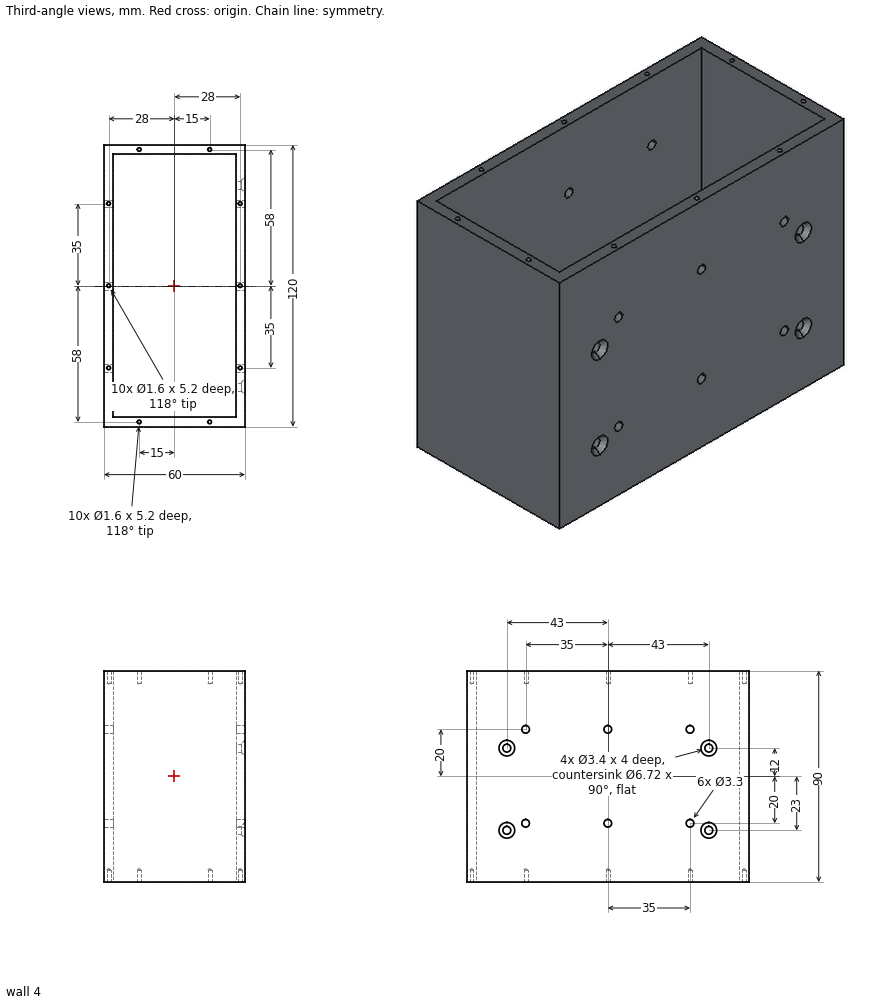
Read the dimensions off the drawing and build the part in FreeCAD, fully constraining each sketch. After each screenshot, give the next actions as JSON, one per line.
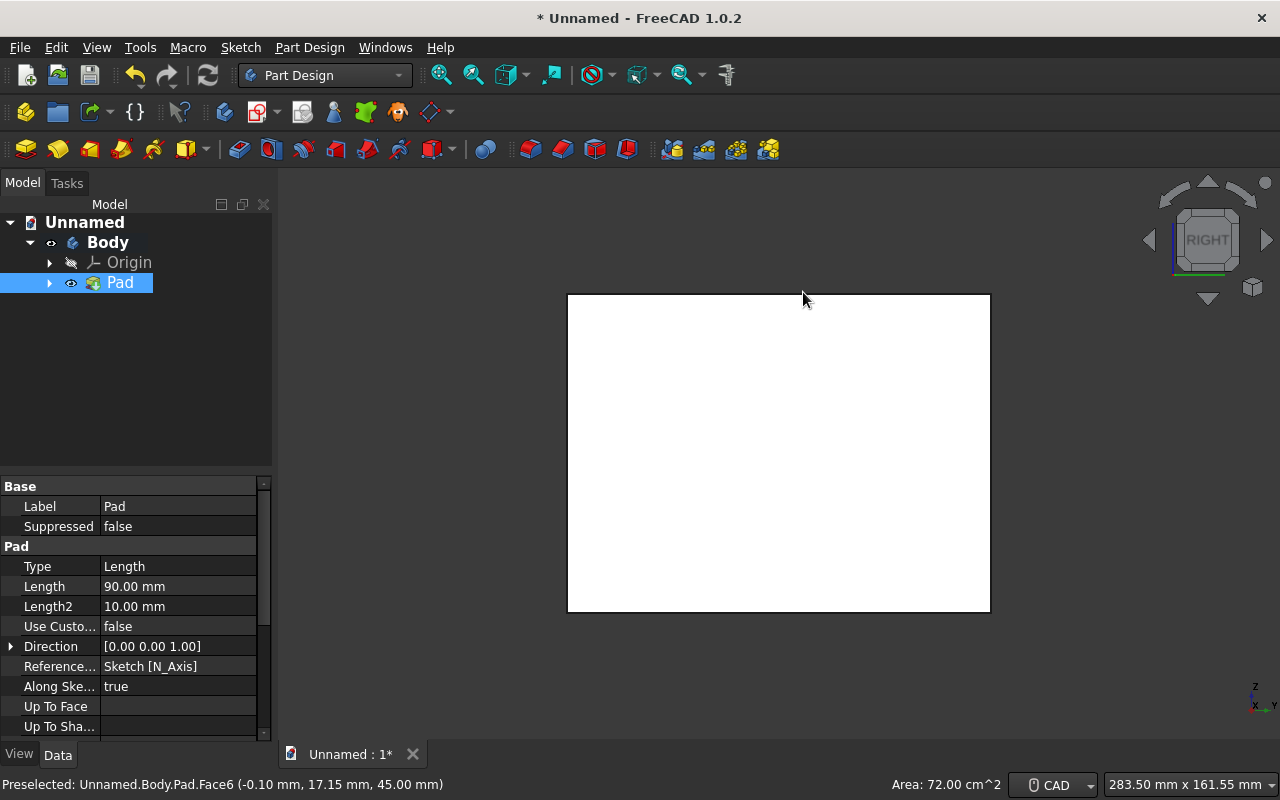
{"action": "key", "text": "5"}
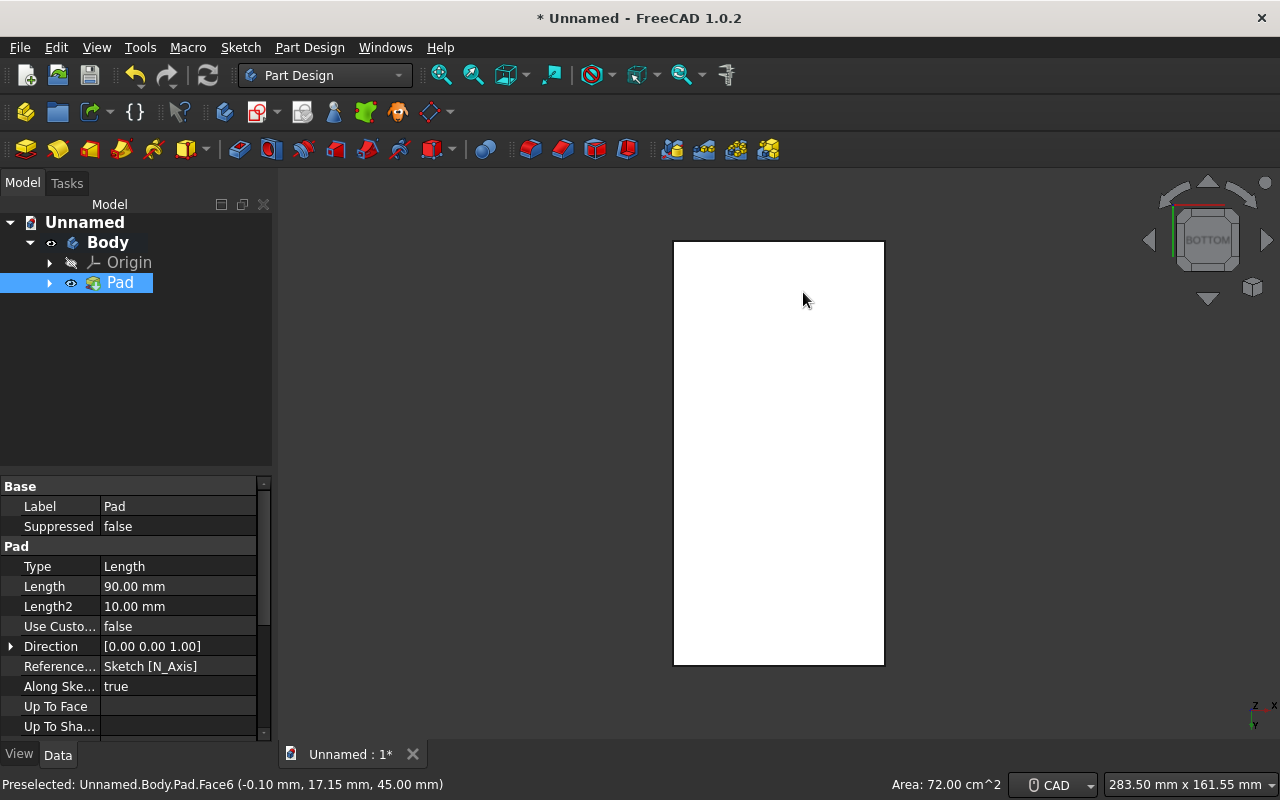
{"action": "left_click", "coordinate": [779, 513], "text": "ctrl"}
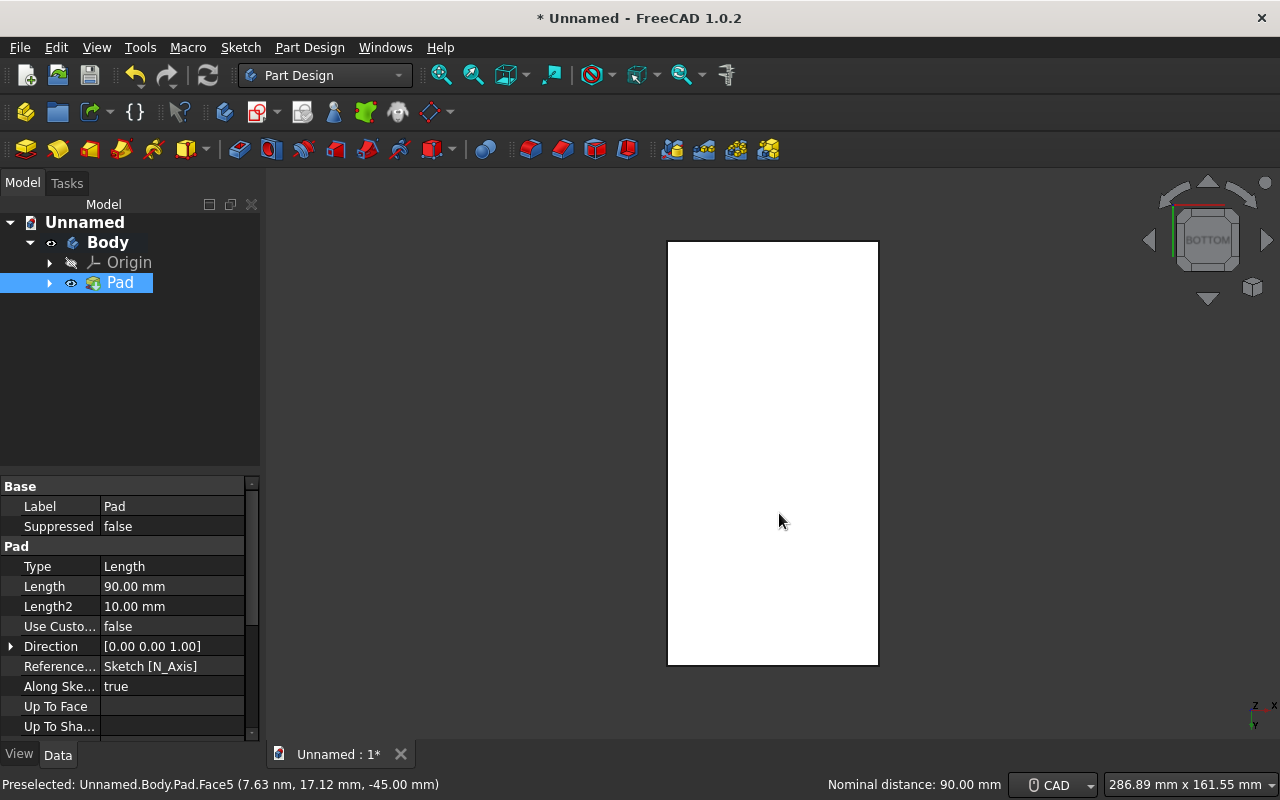
{"action": "left_click", "coordinate": [628, 150]}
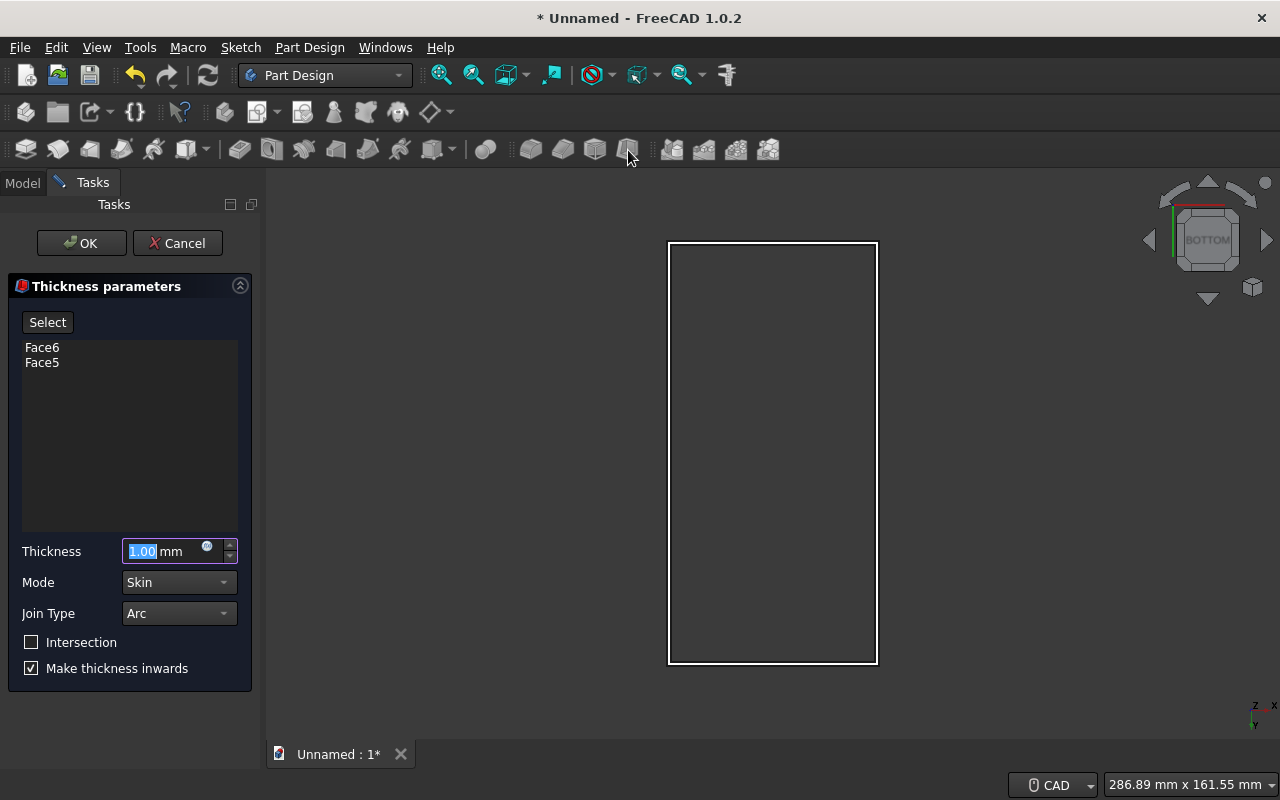
{"action": "type", "text": "4"}
{"action": "key", "text": "Tab"}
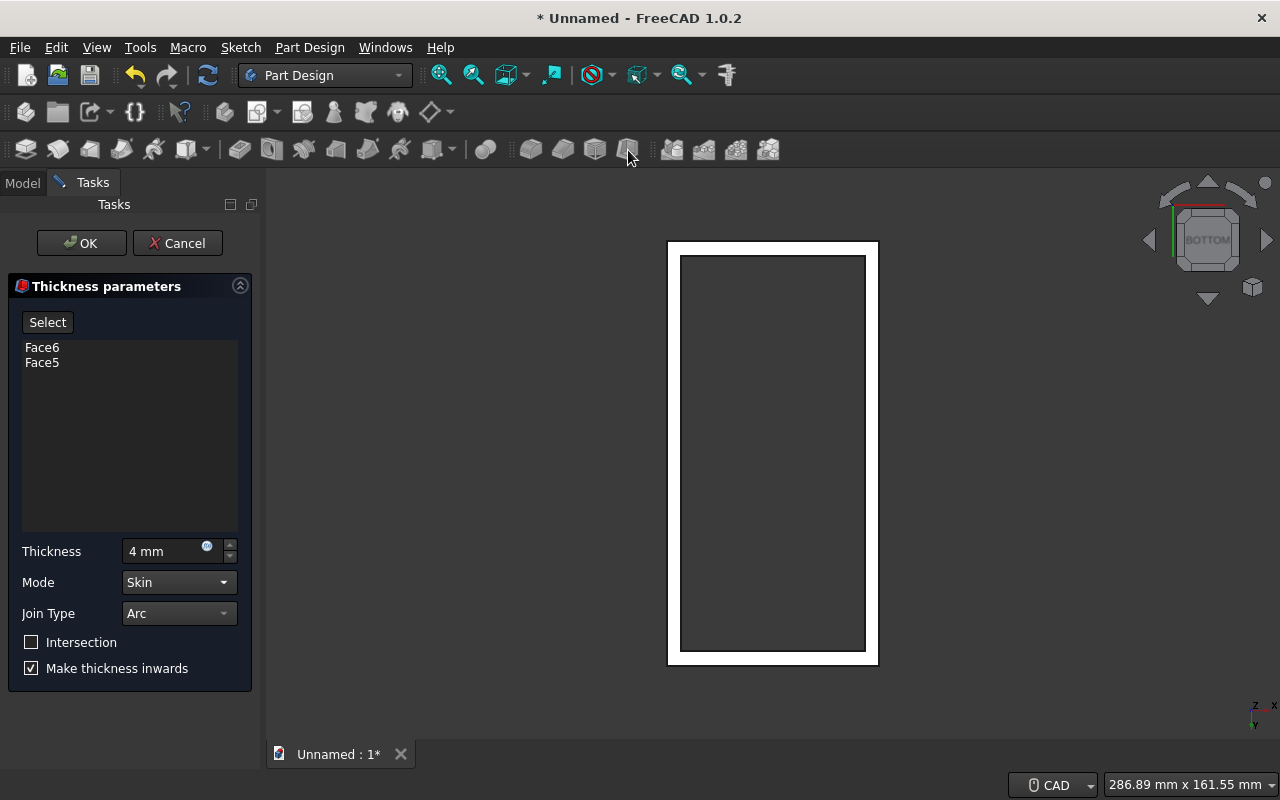
{"action": "left_click", "coordinate": [180, 614]}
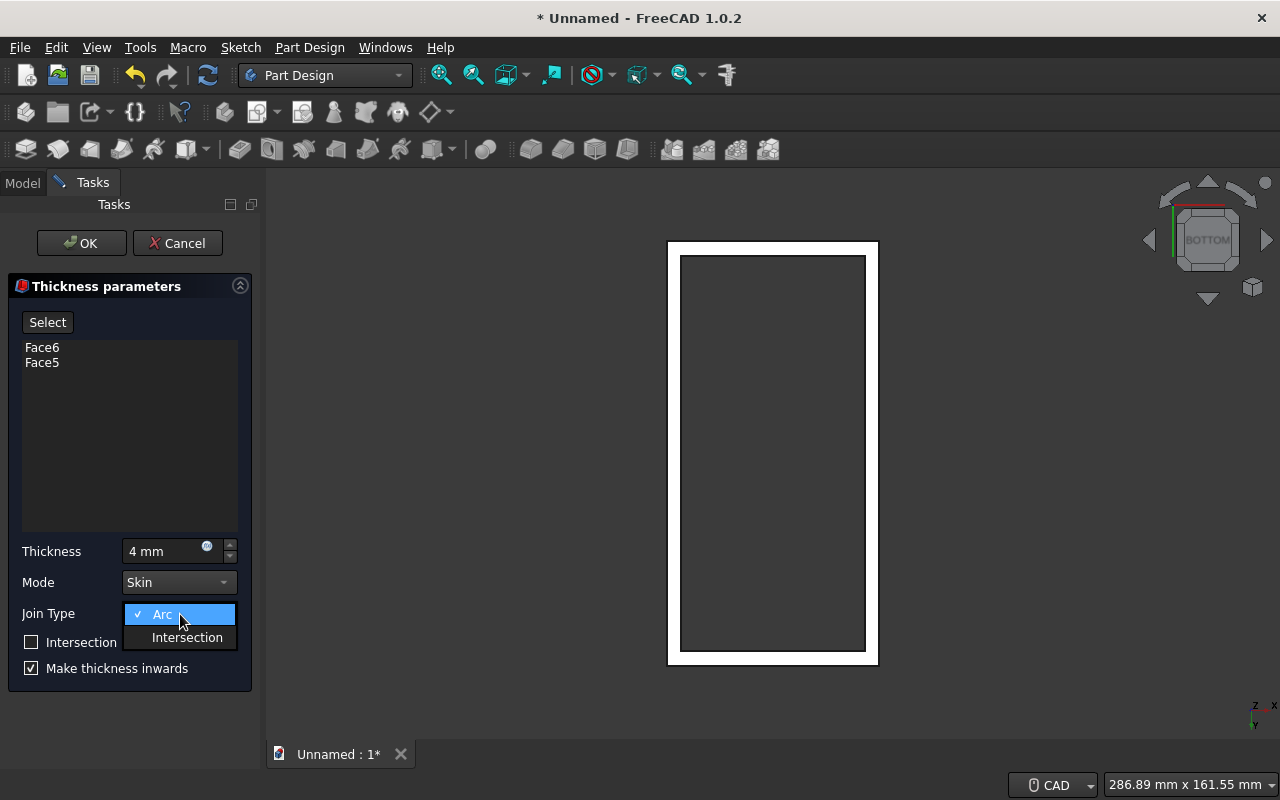
{"action": "left_click", "coordinate": [179, 638]}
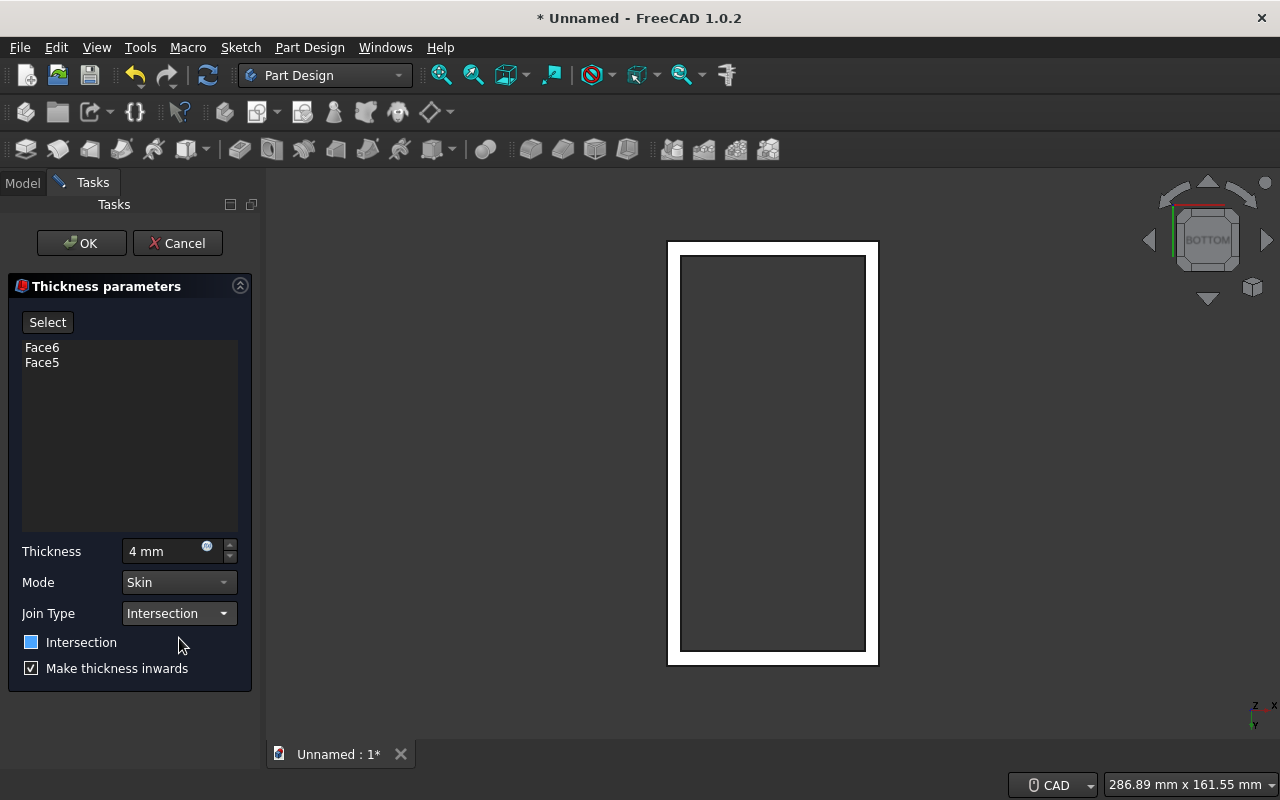
{"action": "left_click", "coordinate": [82, 243]}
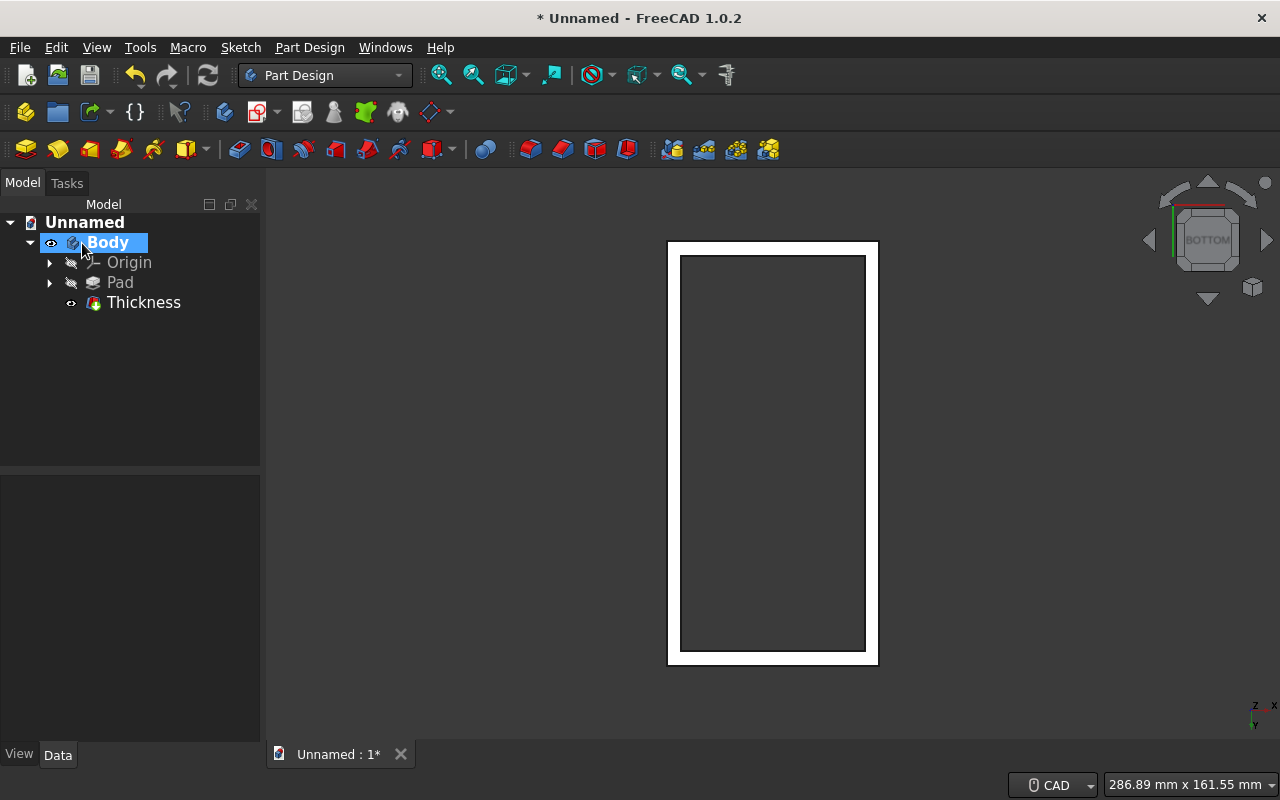
{"action": "key", "text": "0"}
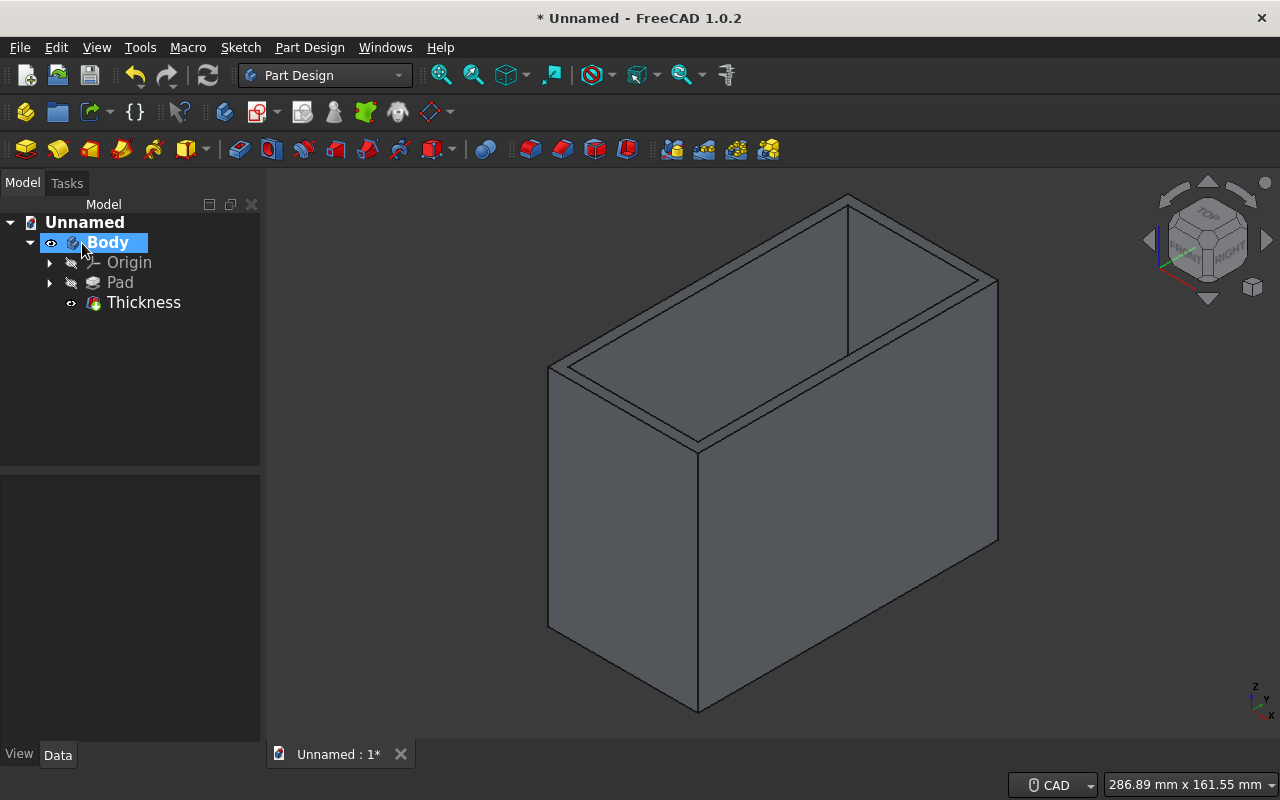
{"action": "scroll", "coordinate": [941, 254], "scroll_direction": "up", "scroll_amount": 5}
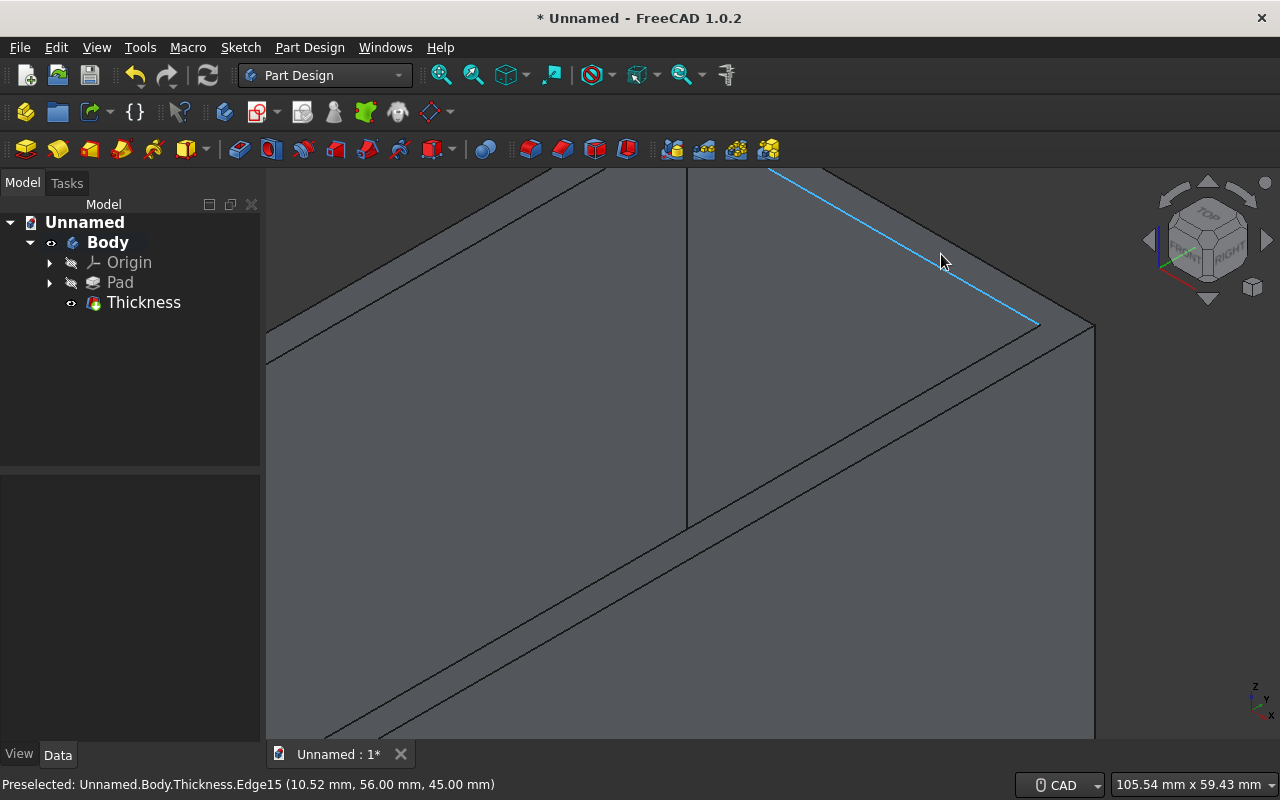
{"action": "left_click", "coordinate": [941, 256]}